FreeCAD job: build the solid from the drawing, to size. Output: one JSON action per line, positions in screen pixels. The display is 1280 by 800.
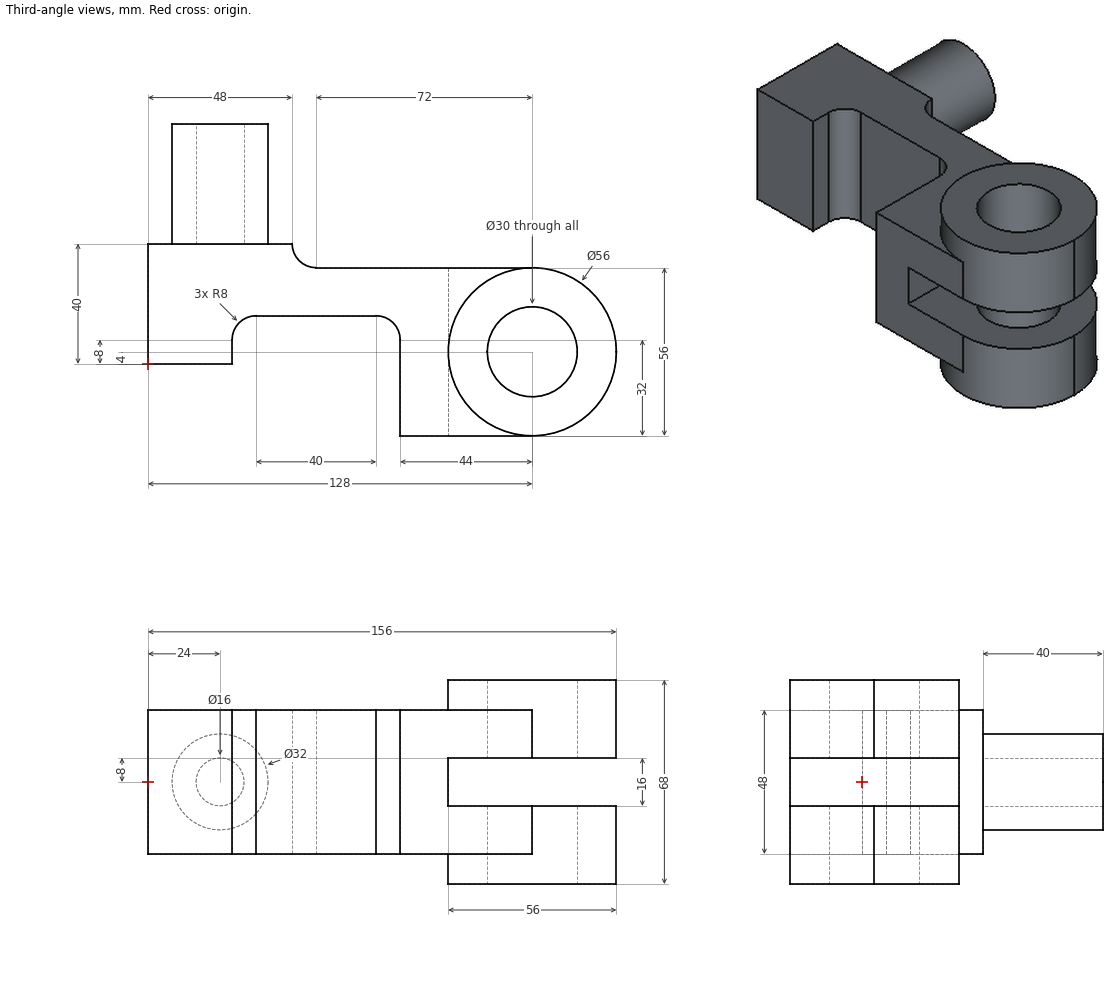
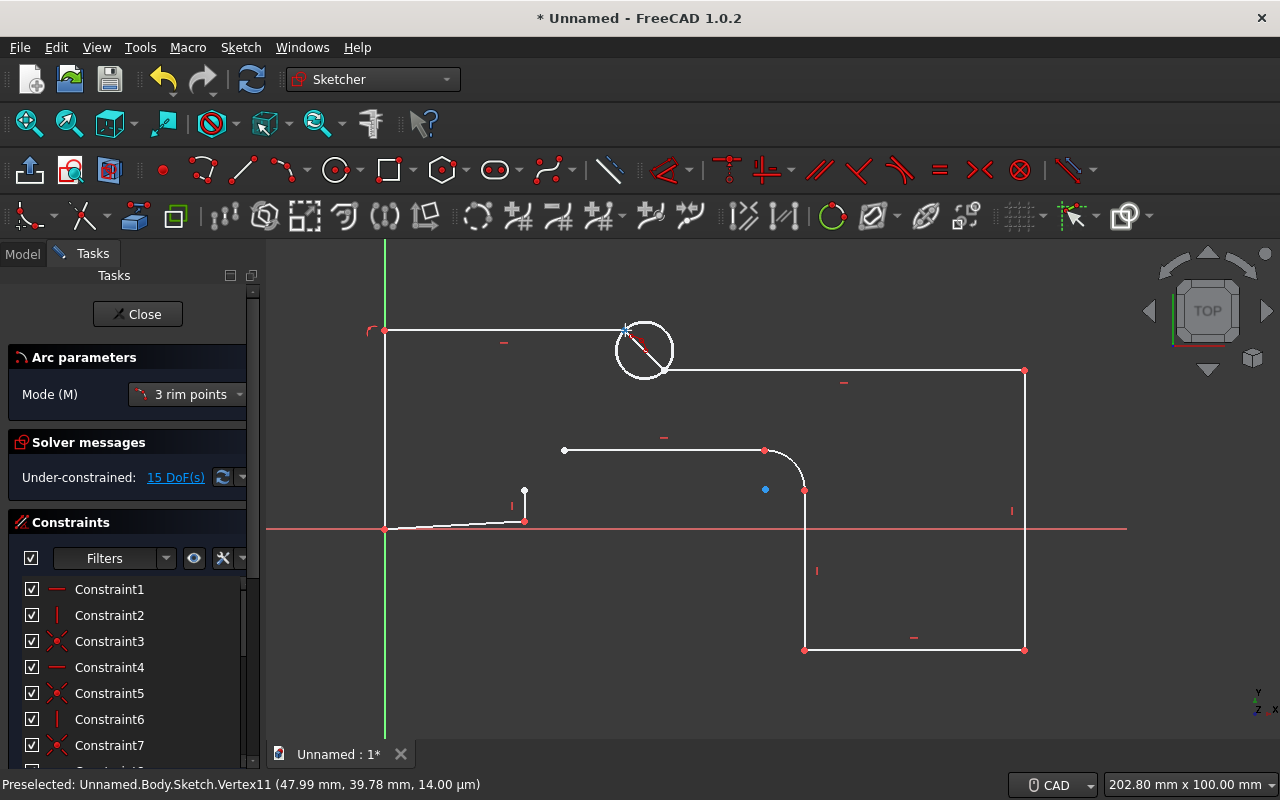
{"action": "scroll", "coordinate": [636, 358], "scroll_direction": "up", "scroll_amount": 2}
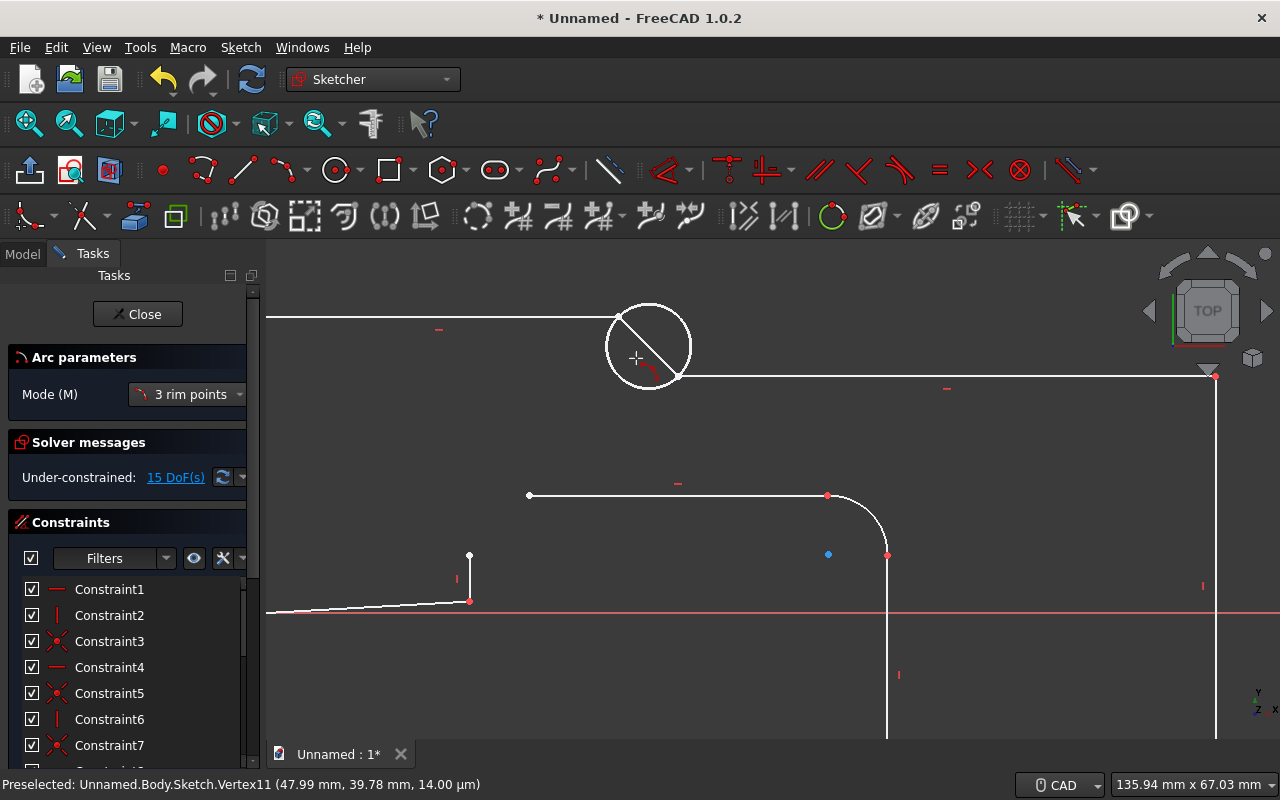
{"action": "left_click", "coordinate": [636, 357]}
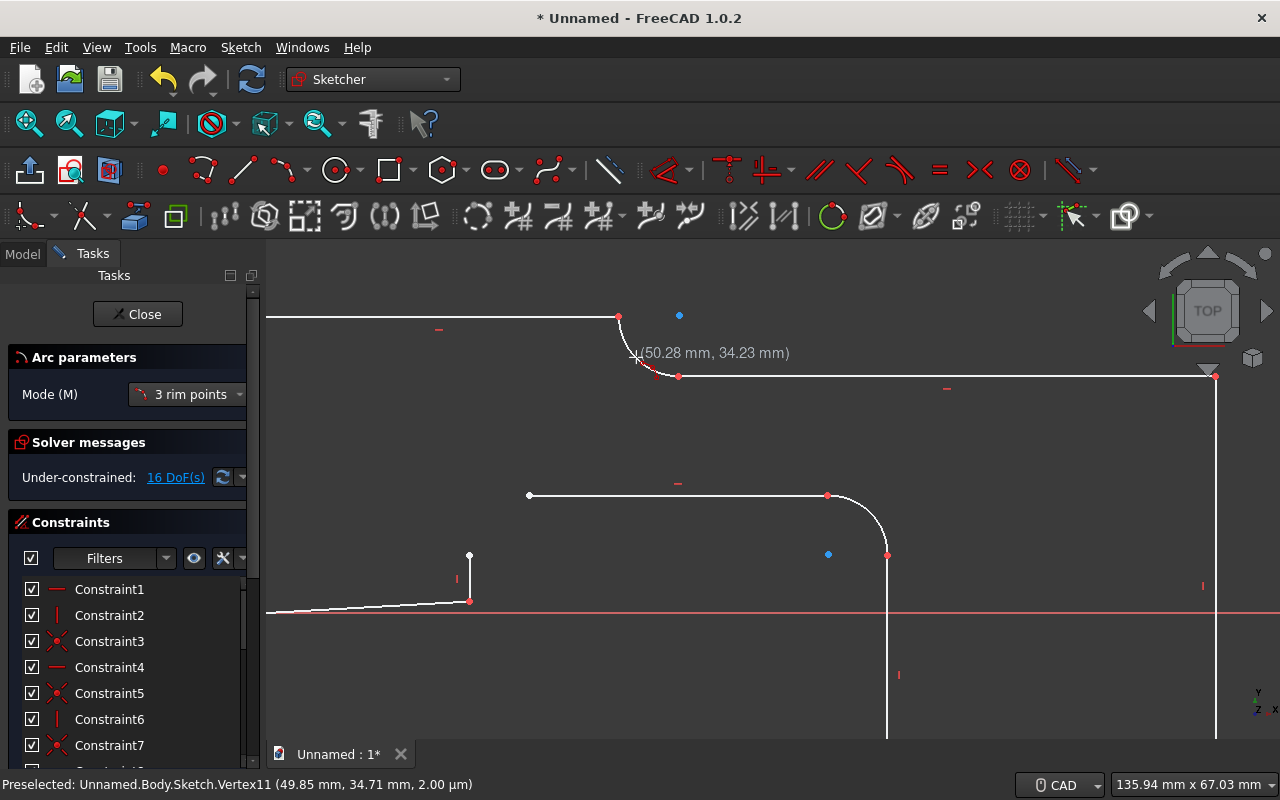
{"action": "left_click", "coordinate": [470, 555]}
{"action": "left_click", "coordinate": [529, 496]}
{"action": "left_click", "coordinate": [487, 511]}
{"action": "key", "text": "Escape"}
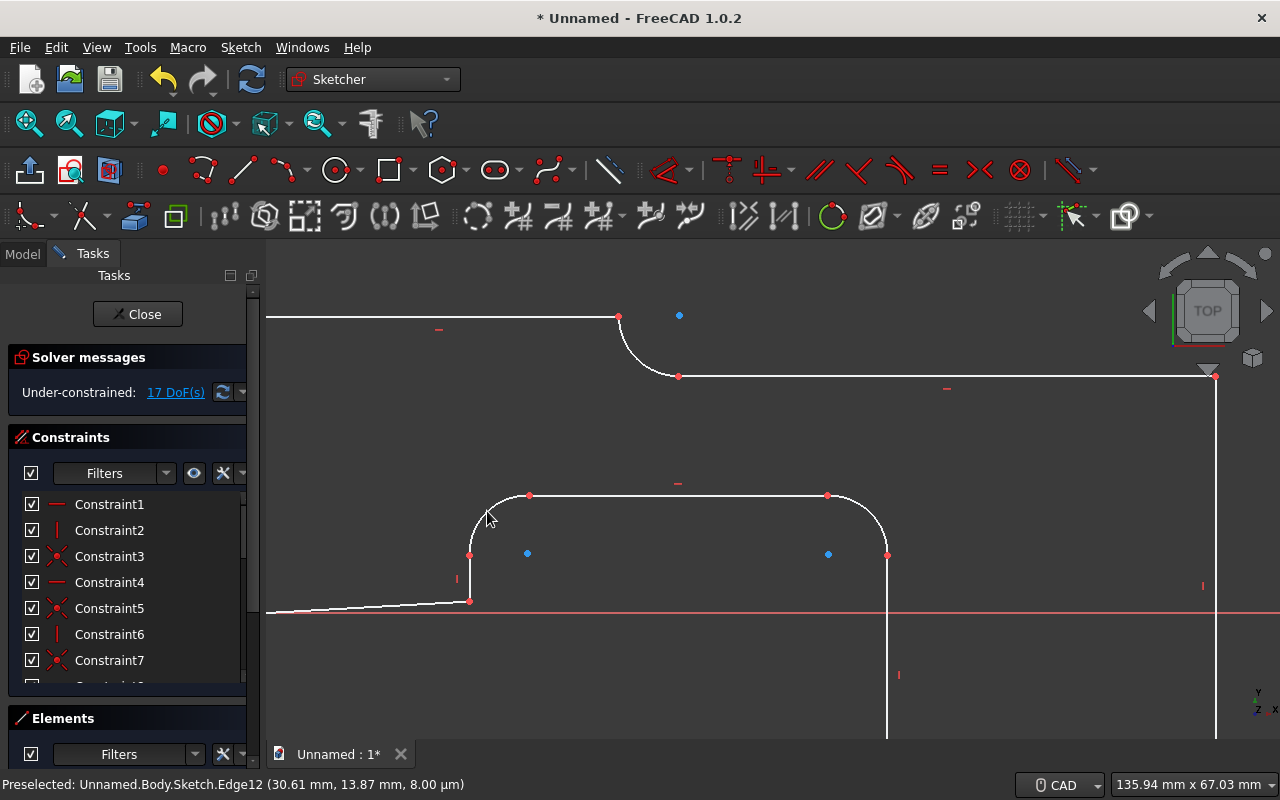
{"action": "left_click", "coordinate": [619, 496]}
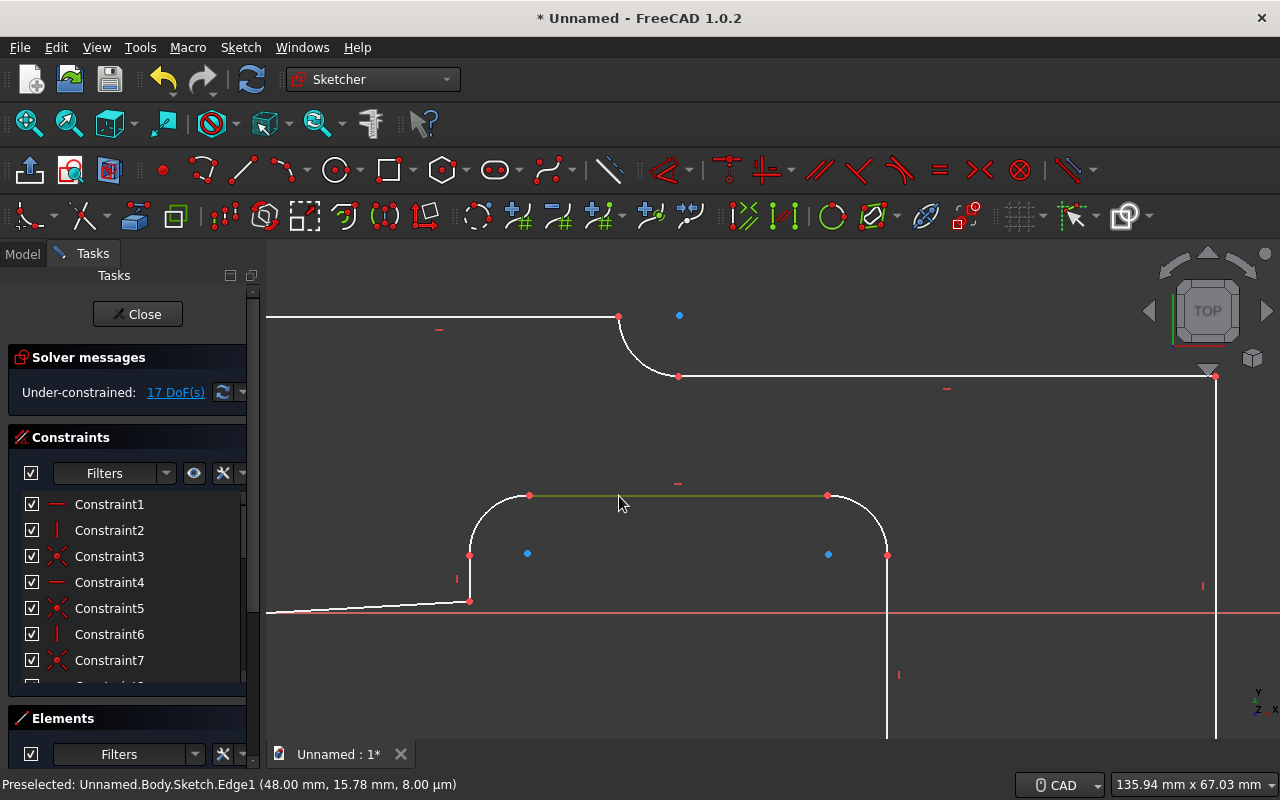
{"action": "left_click", "coordinate": [881, 528]}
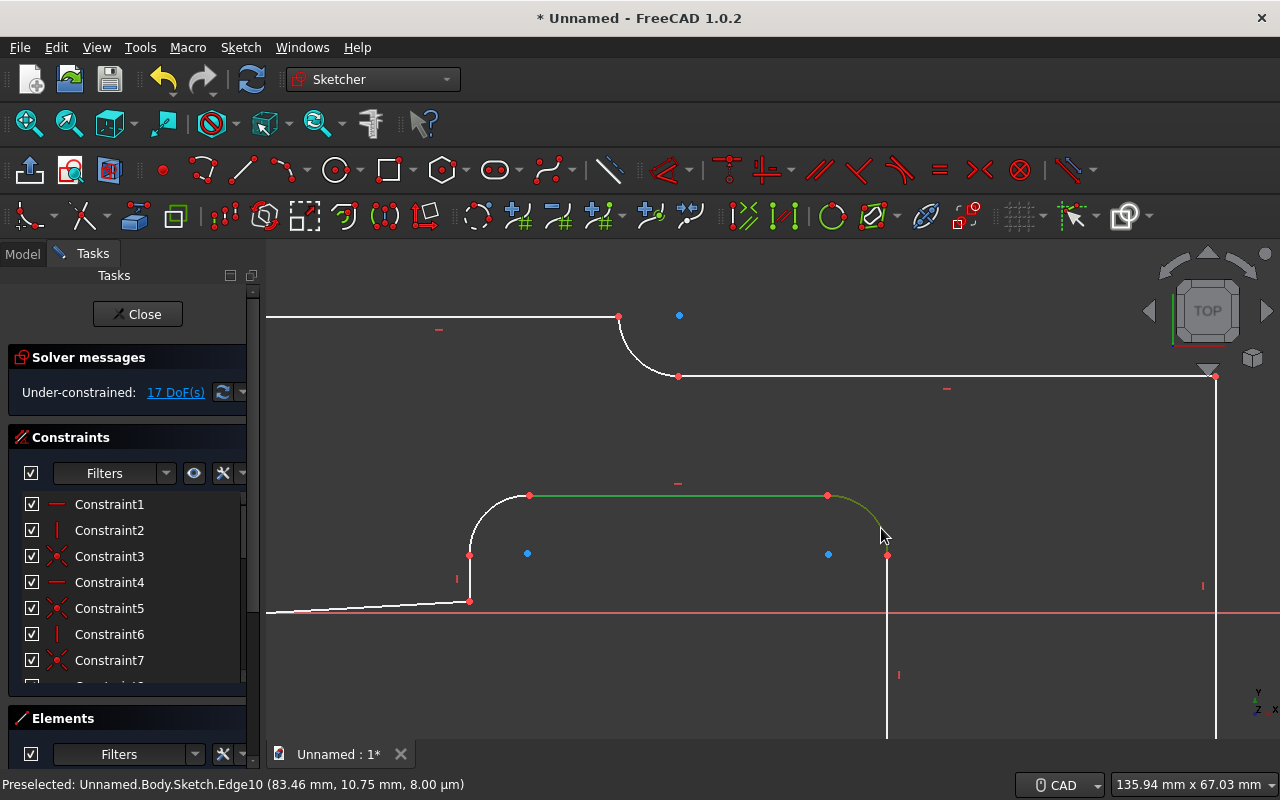
{"action": "key", "text": "t"}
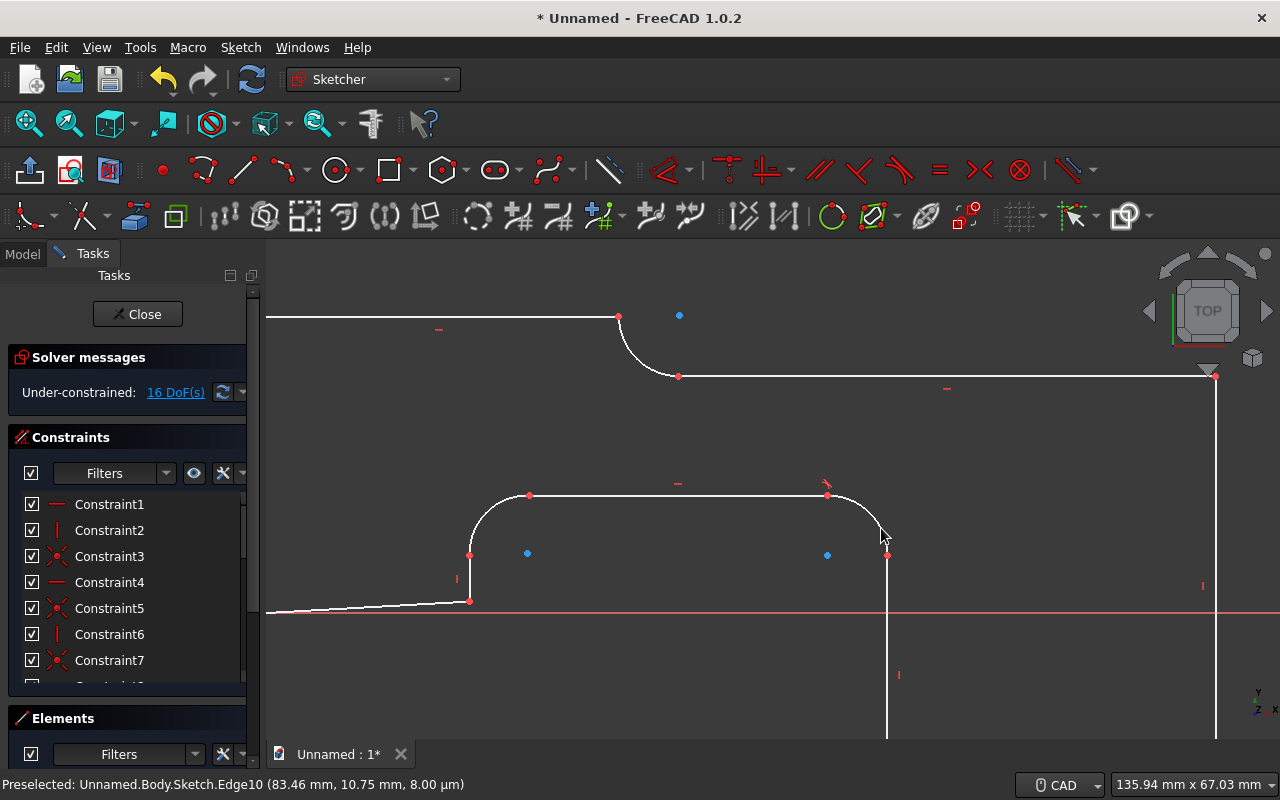
{"action": "left_click", "coordinate": [619, 496]}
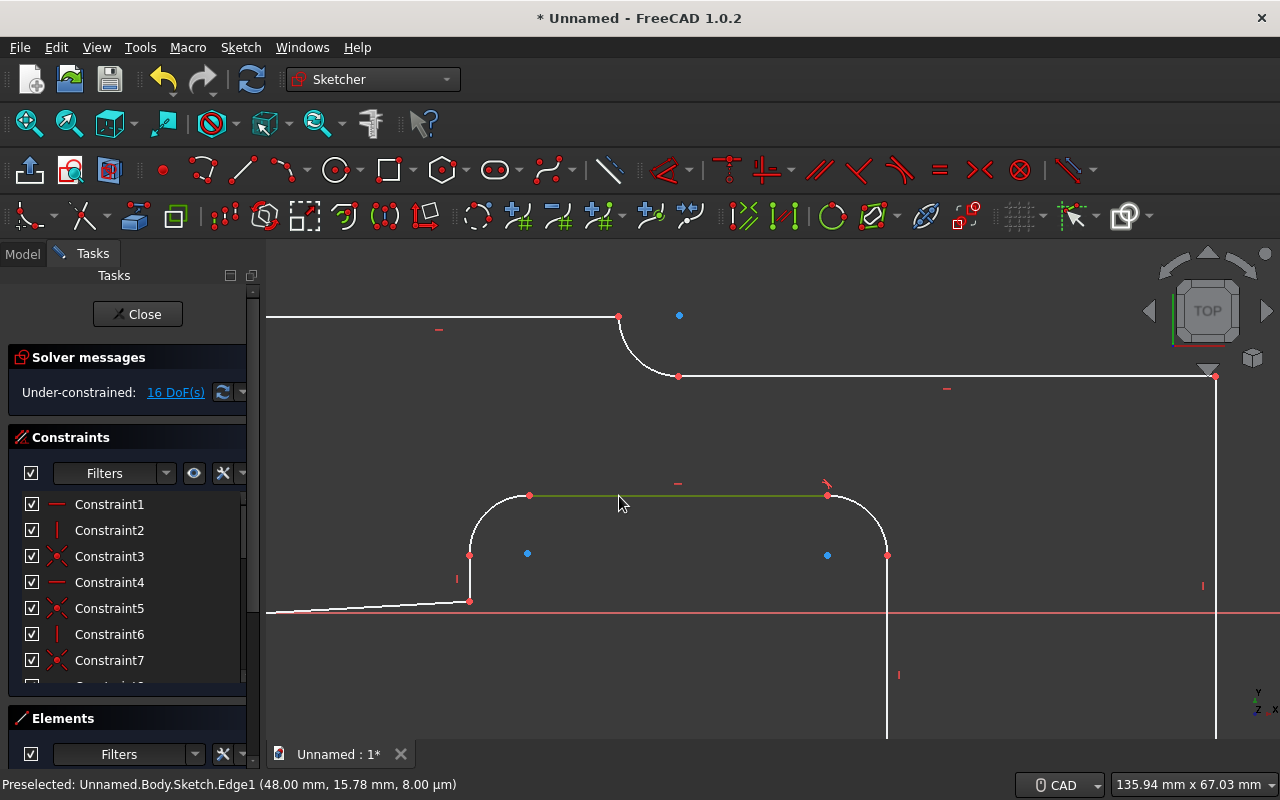
{"action": "left_click", "coordinate": [502, 501]}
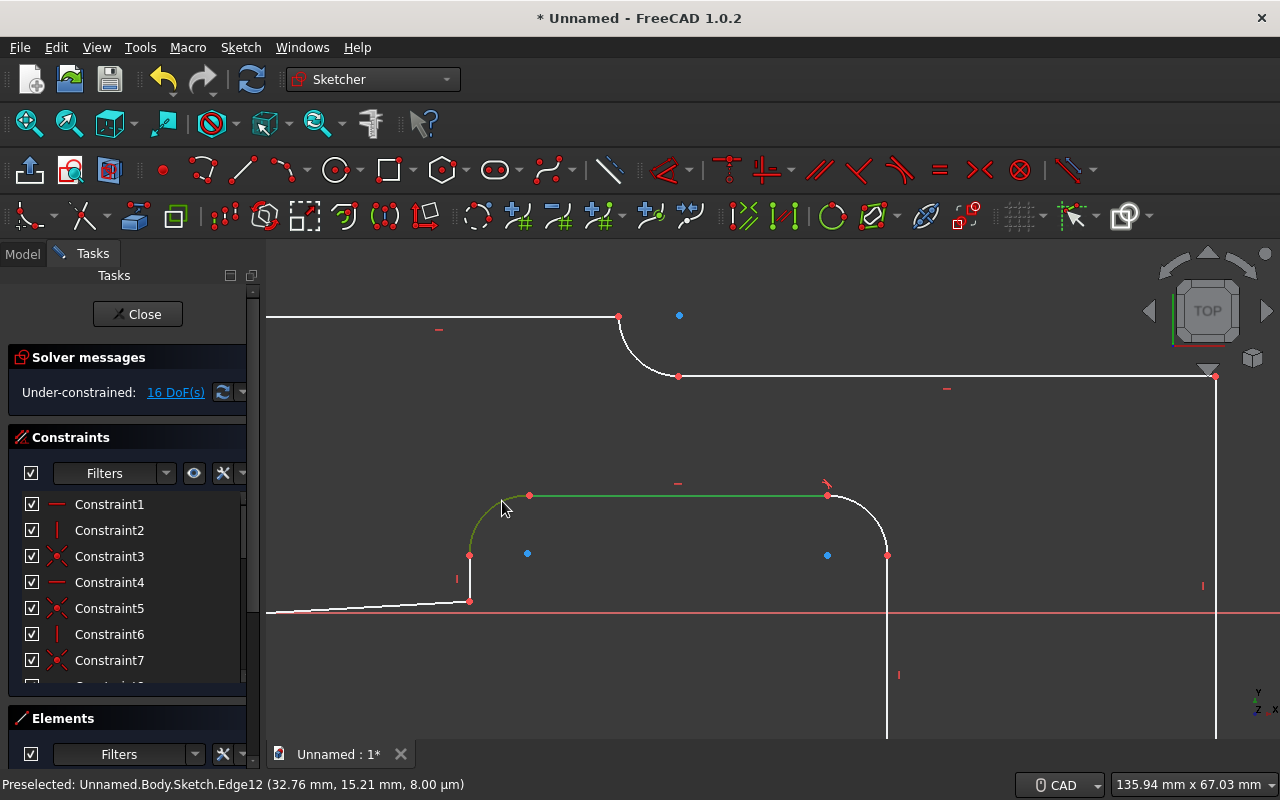
{"action": "key", "text": "t"}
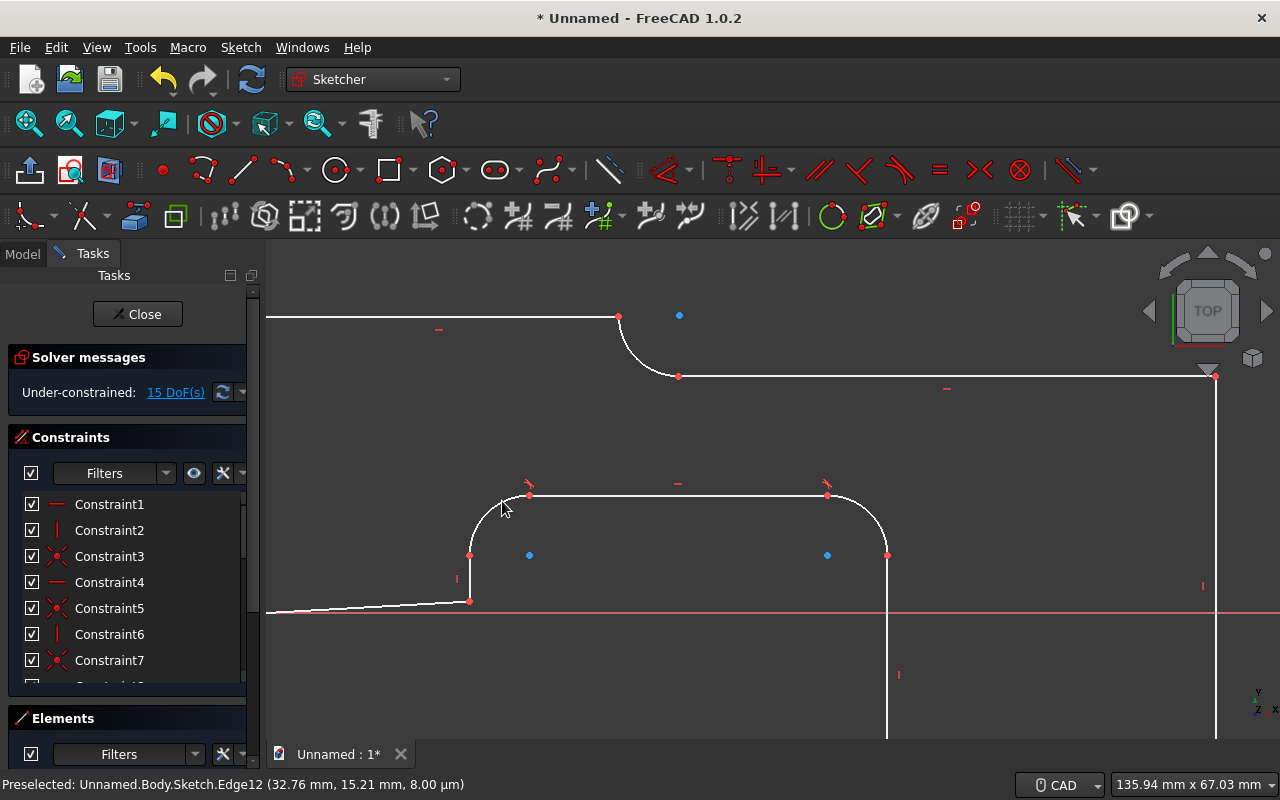
{"action": "left_click", "coordinate": [887, 627]}